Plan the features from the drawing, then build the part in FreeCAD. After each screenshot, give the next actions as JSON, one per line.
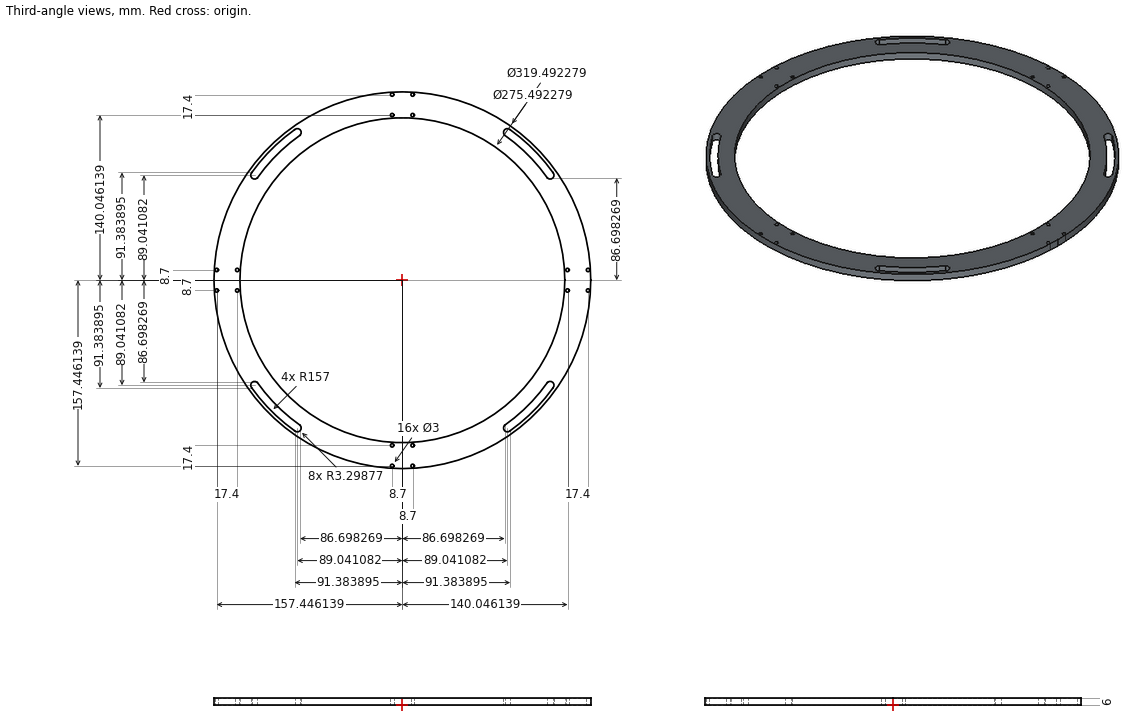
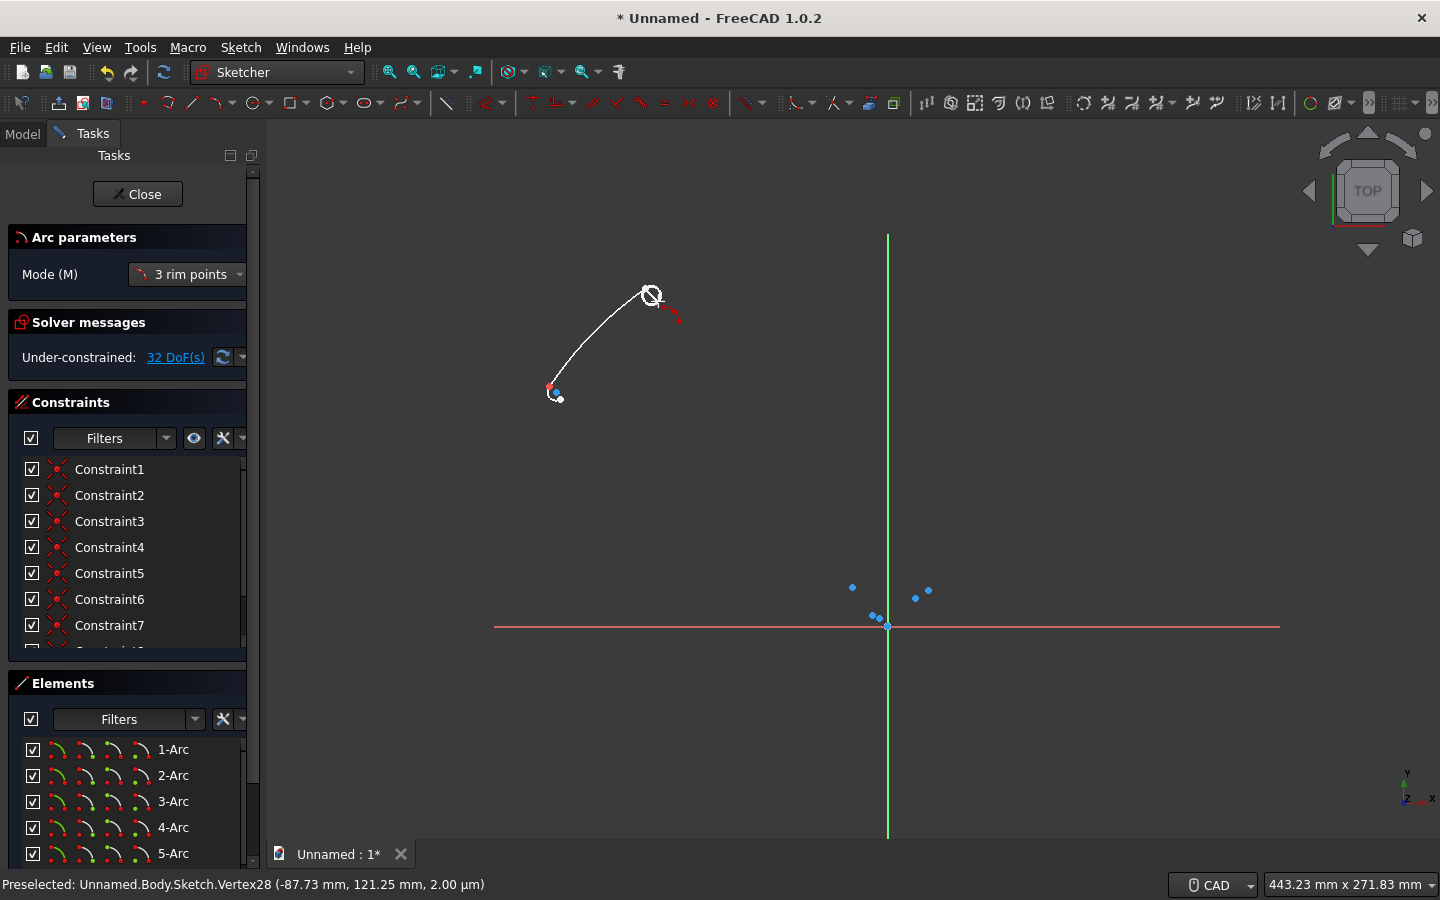
{"action": "scroll", "coordinate": [658, 288], "scroll_direction": "up", "scroll_amount": 3}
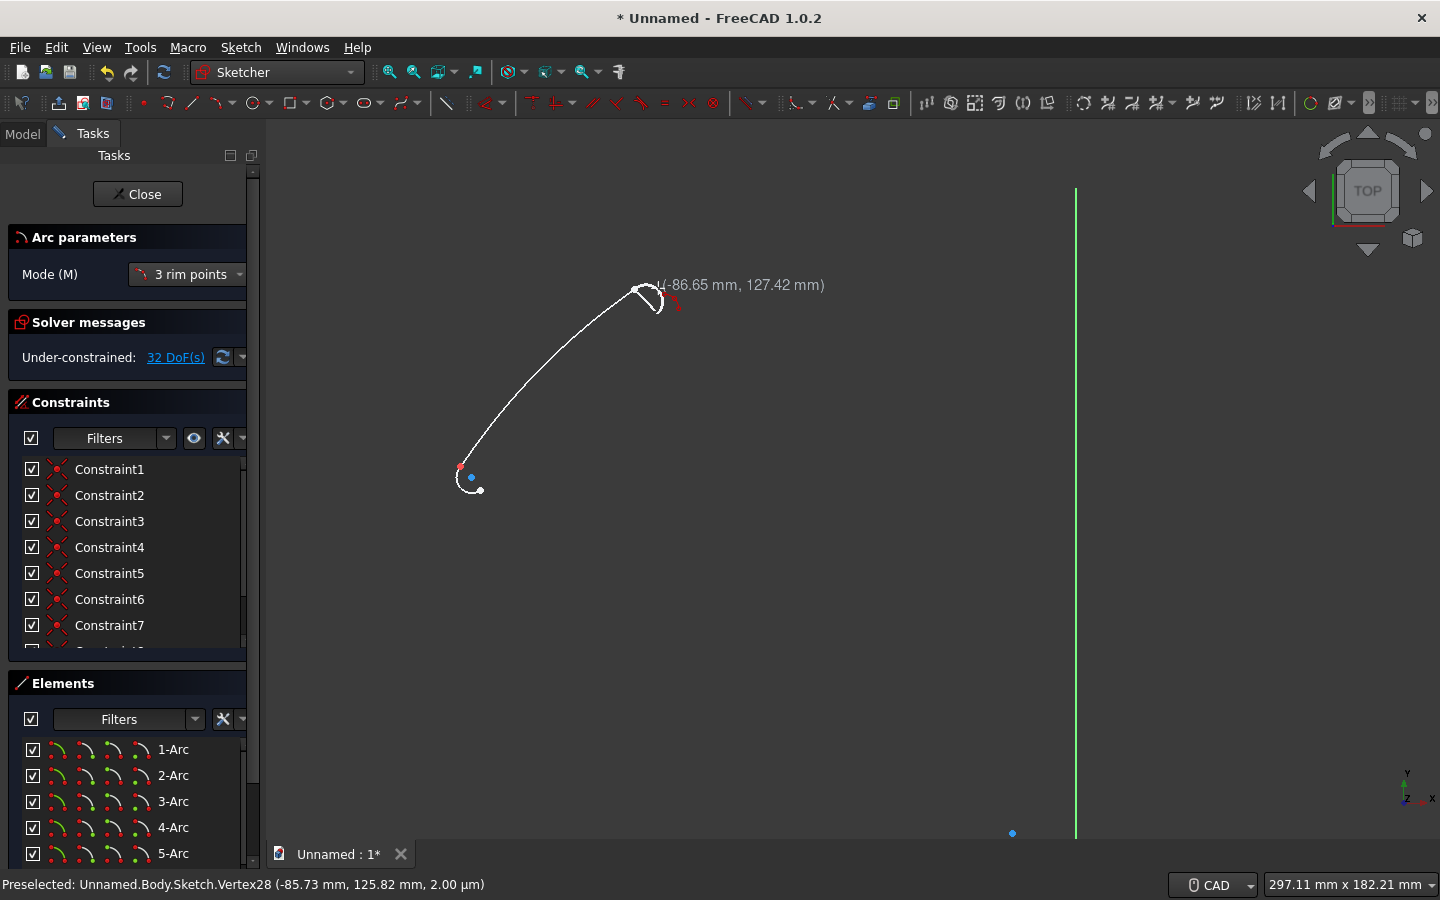
{"action": "left_click", "coordinate": [657, 288]}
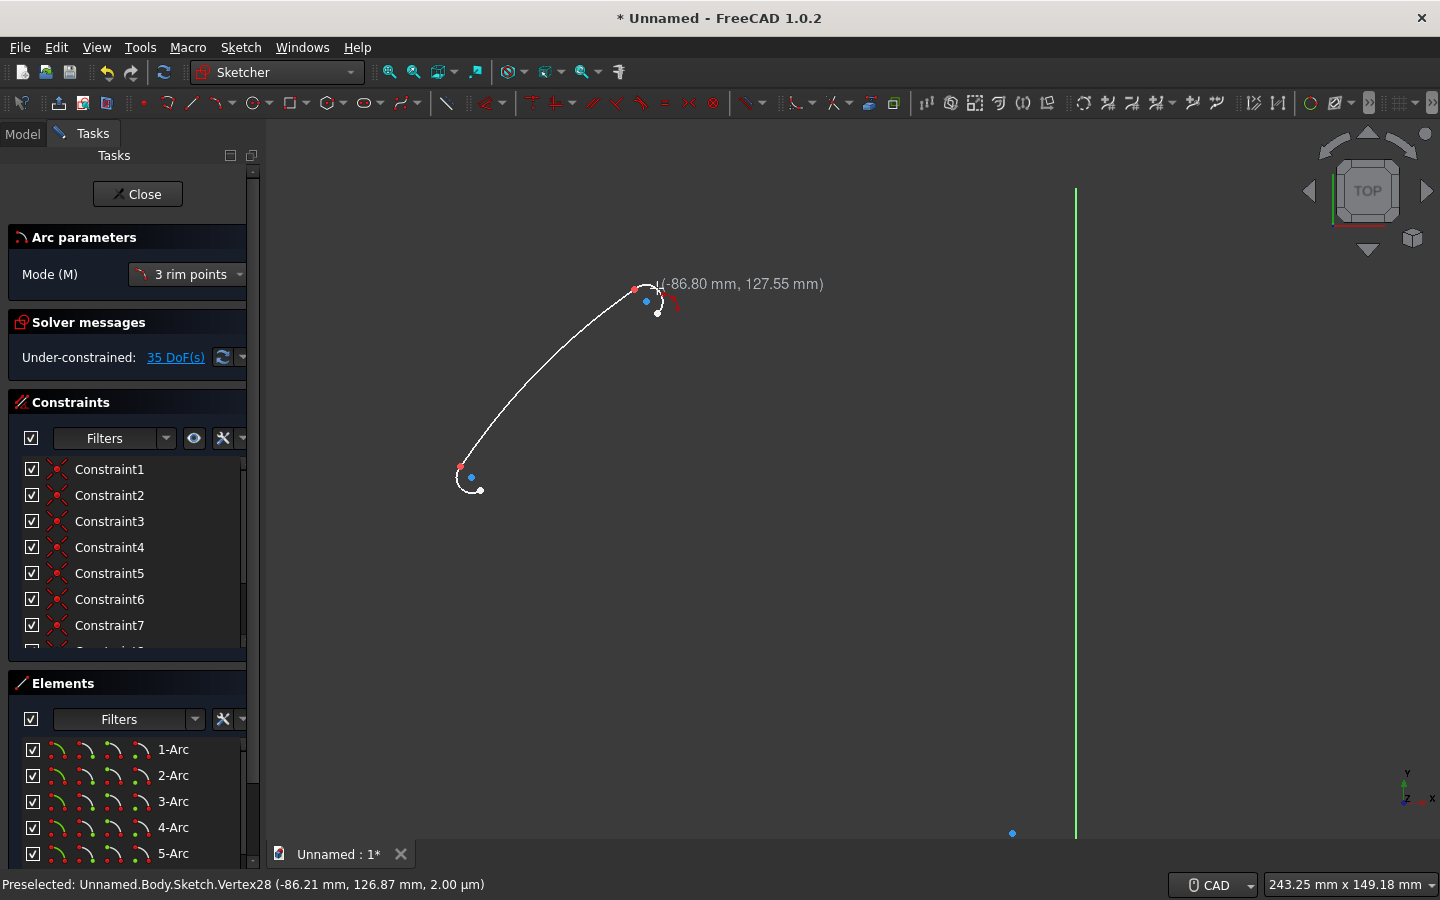
{"action": "left_click", "coordinate": [658, 313]}
{"action": "left_click", "coordinate": [481, 490]}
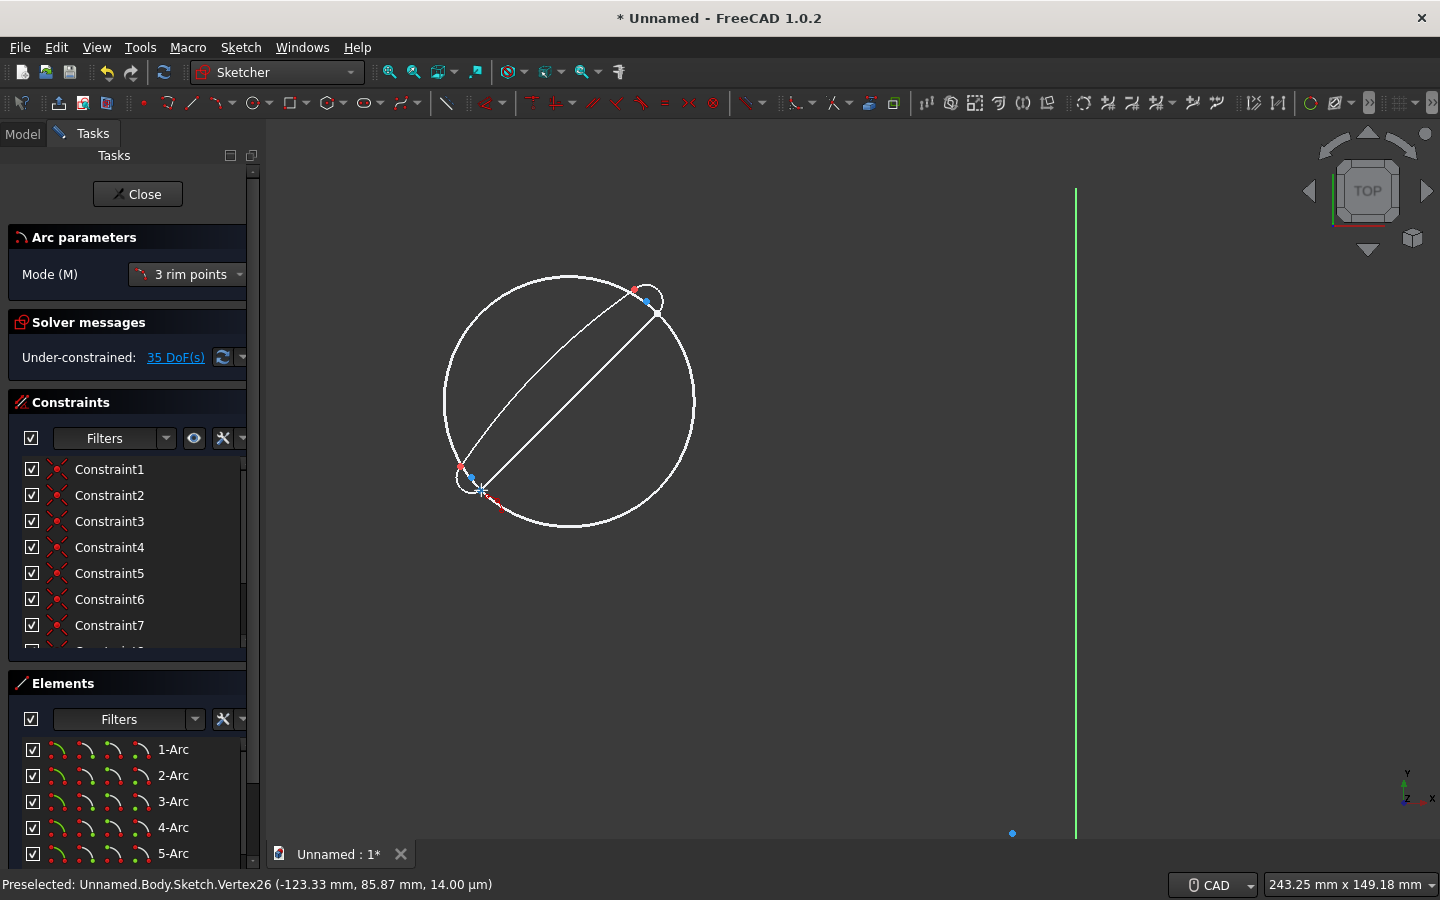
{"action": "scroll", "coordinate": [562, 391], "scroll_direction": "up", "scroll_amount": 2}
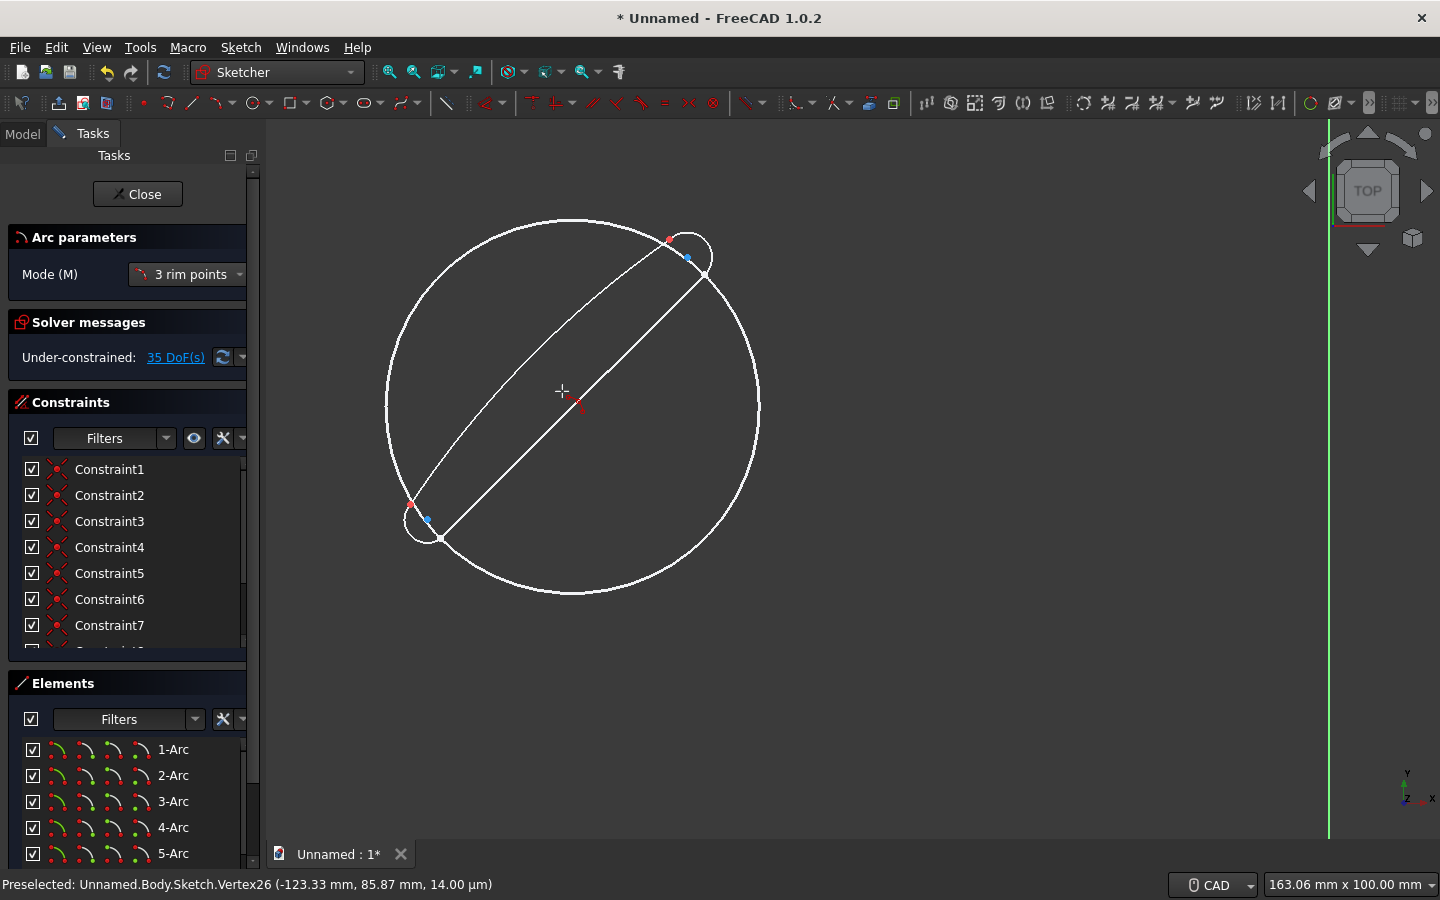
{"action": "left_click", "coordinate": [562, 391]}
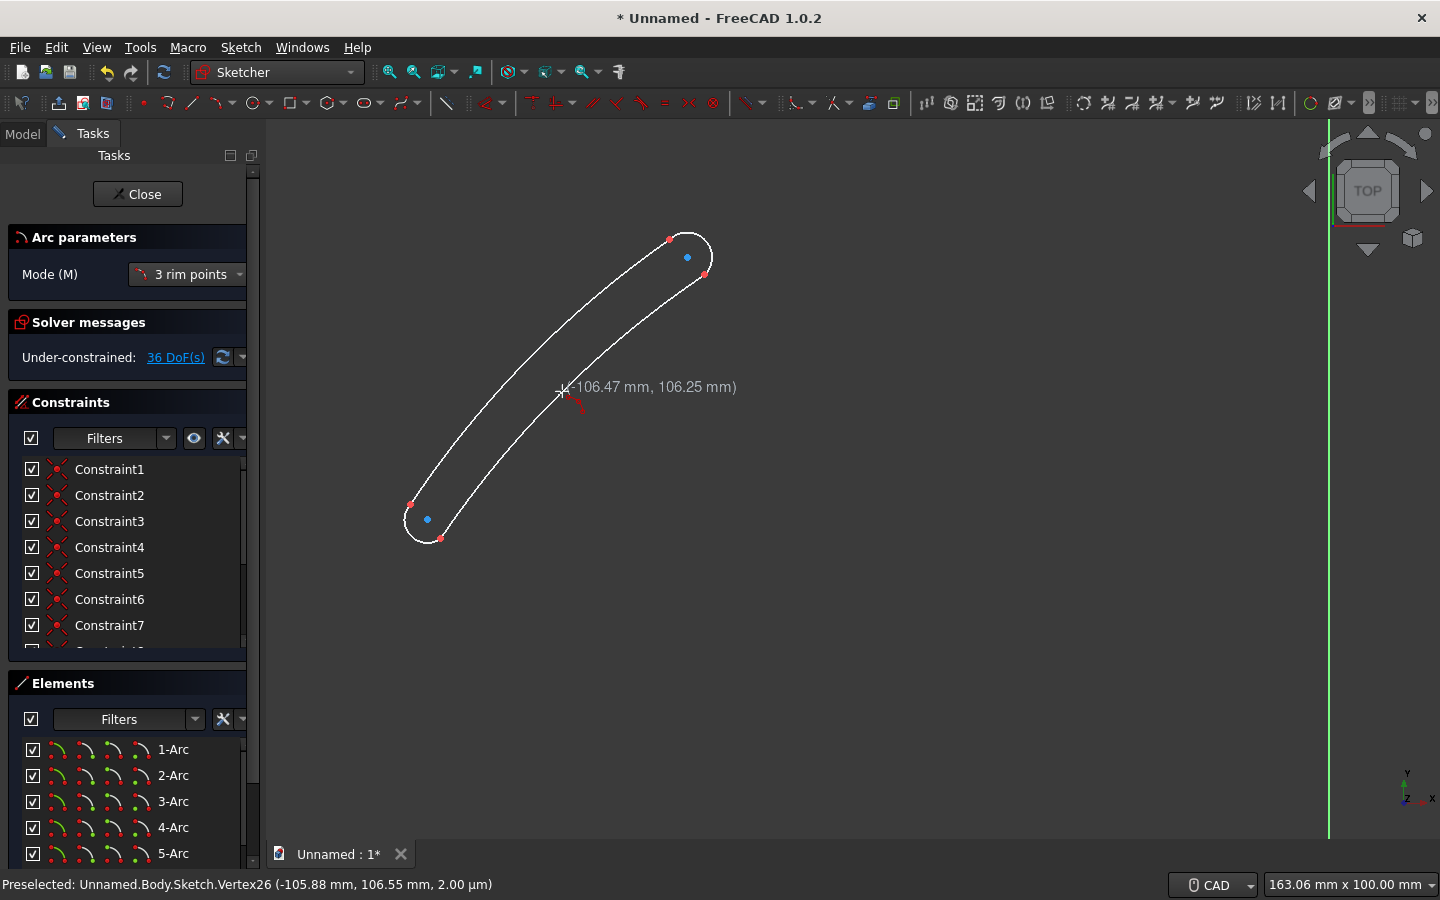
{"action": "scroll", "coordinate": [647, 307], "scroll_direction": "down", "scroll_amount": 8}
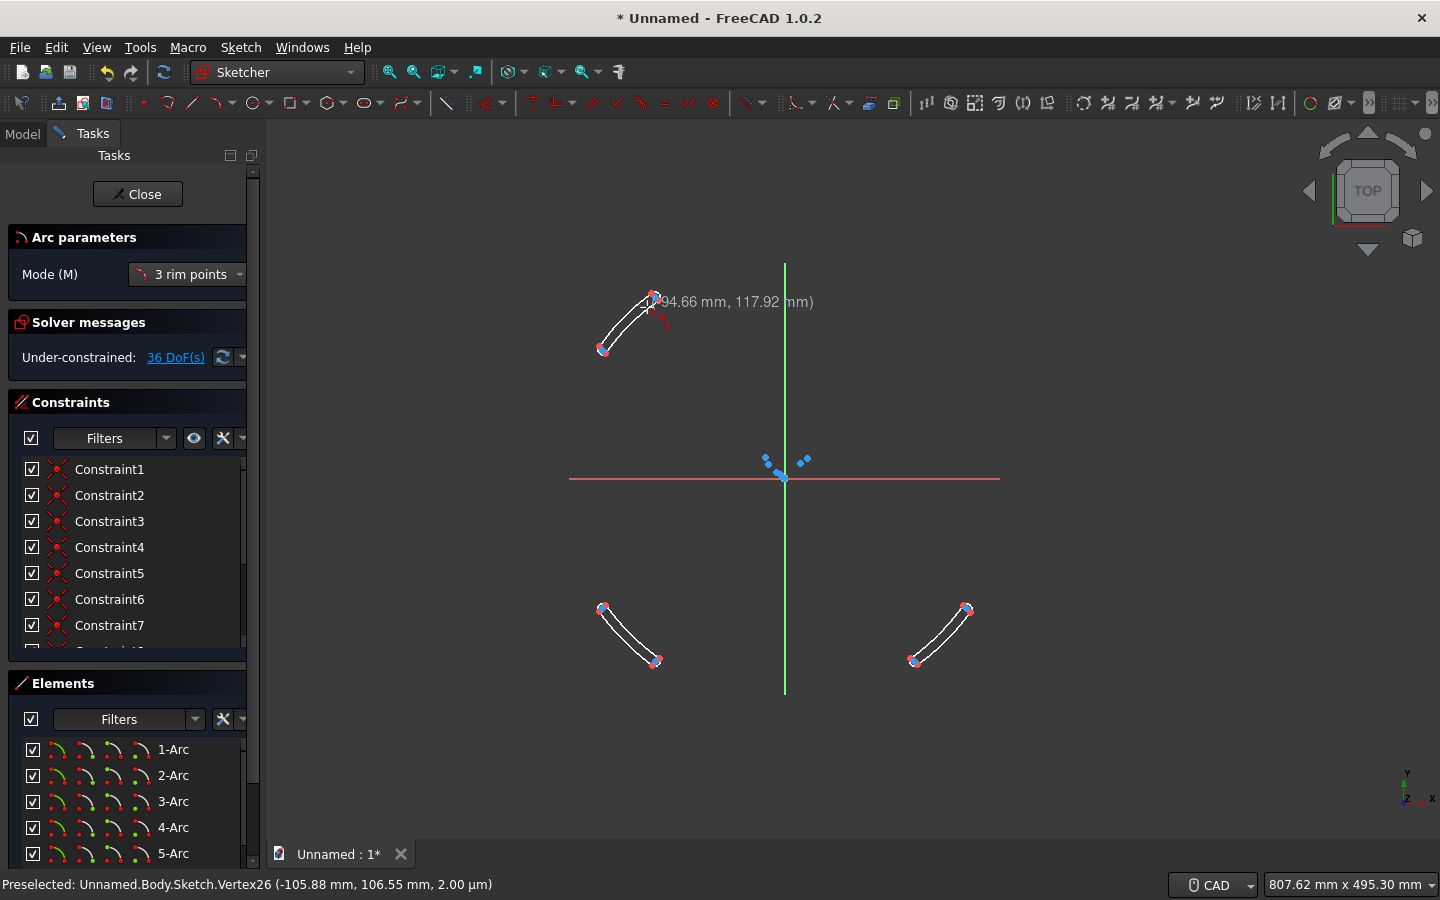
{"action": "left_click", "coordinate": [911, 300]}
{"action": "left_click", "coordinate": [918, 293]}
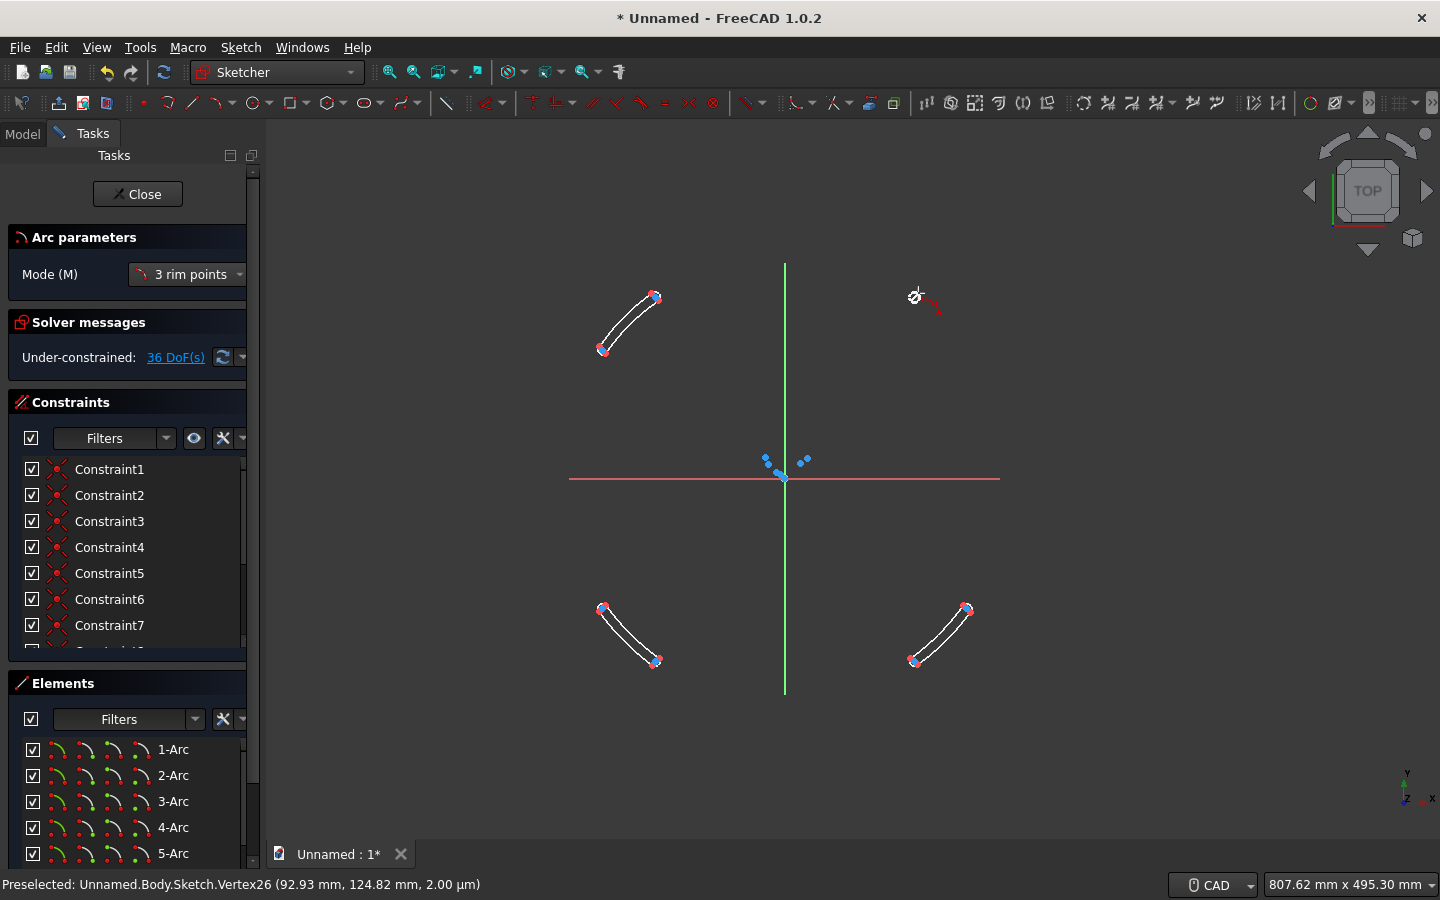
{"action": "scroll", "coordinate": [911, 293], "scroll_direction": "up", "scroll_amount": 6}